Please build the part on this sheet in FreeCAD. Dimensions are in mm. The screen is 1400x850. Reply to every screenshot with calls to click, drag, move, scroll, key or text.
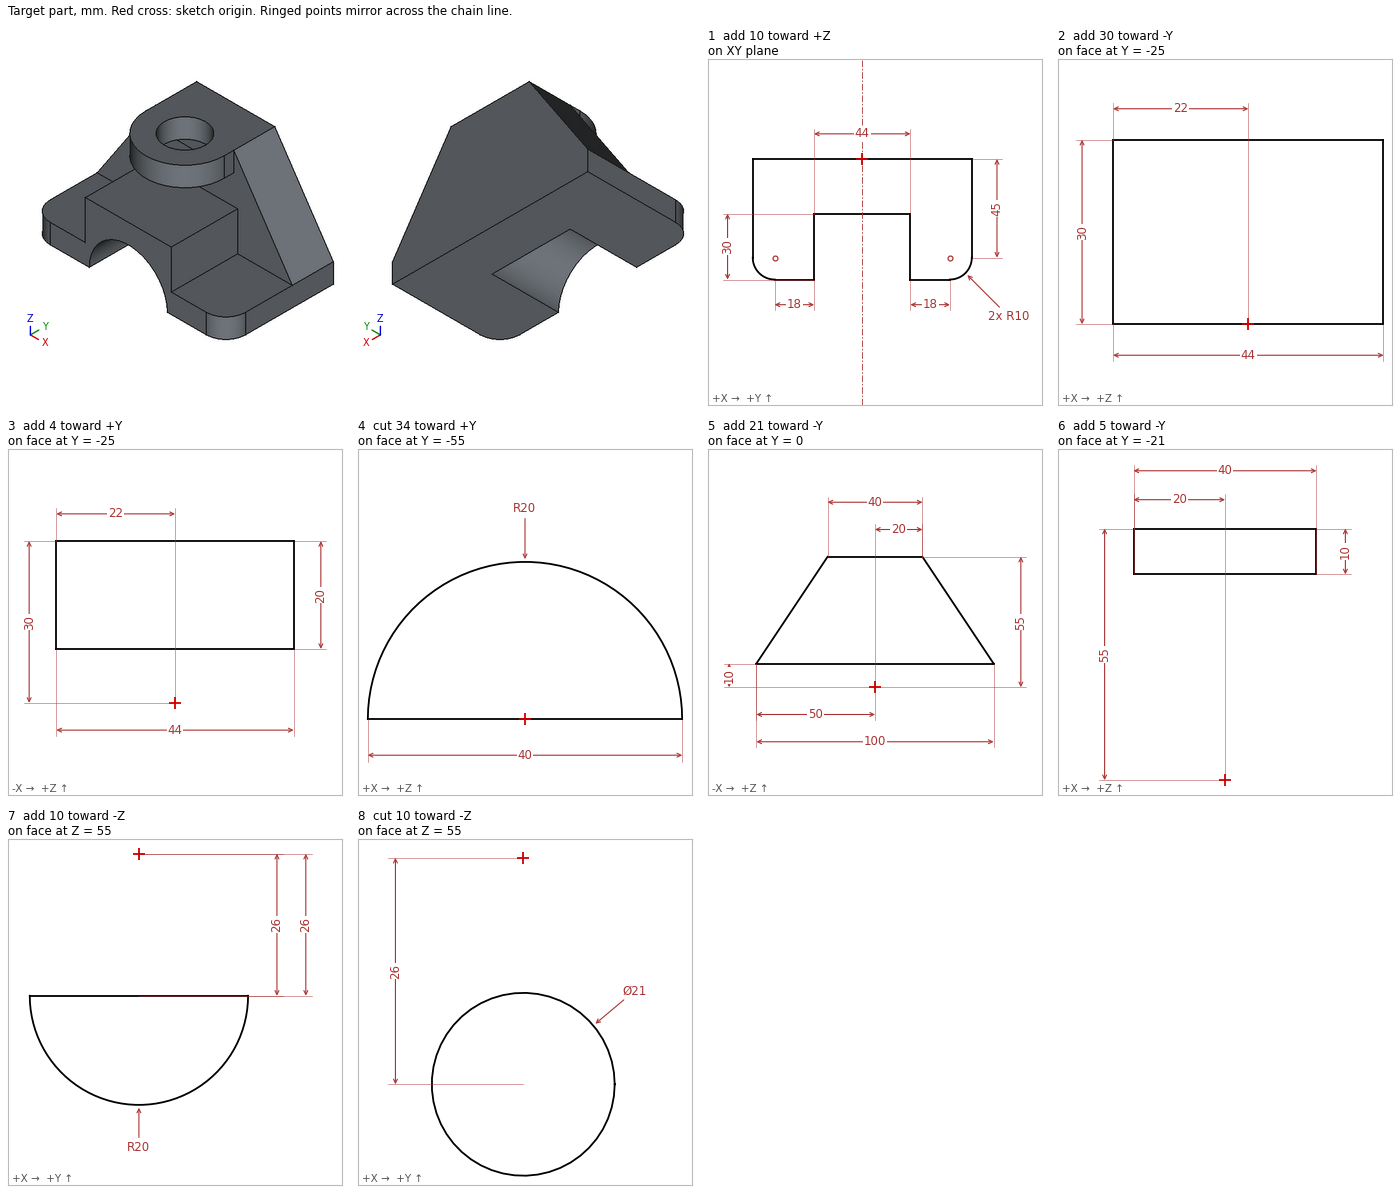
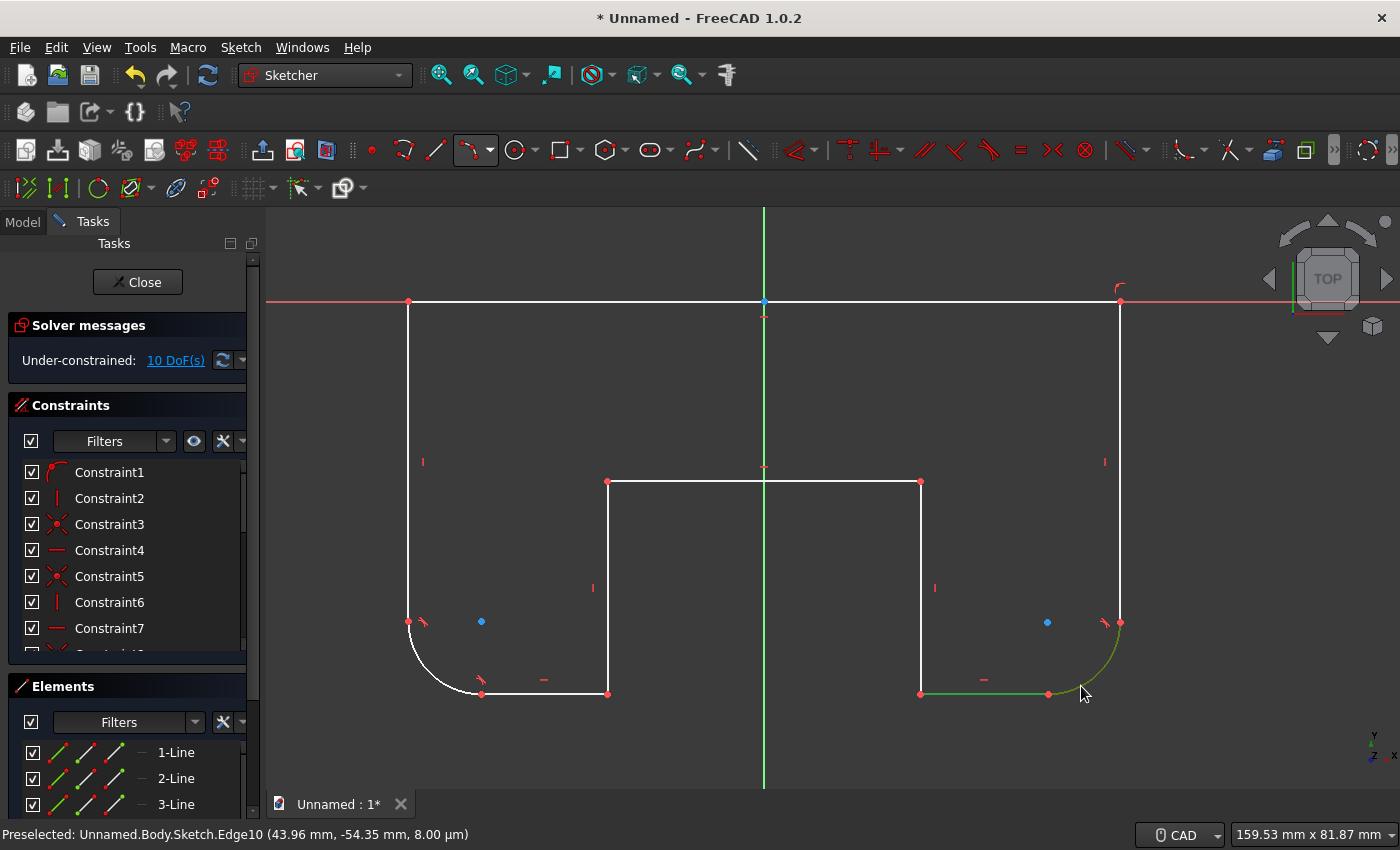
click(990, 150)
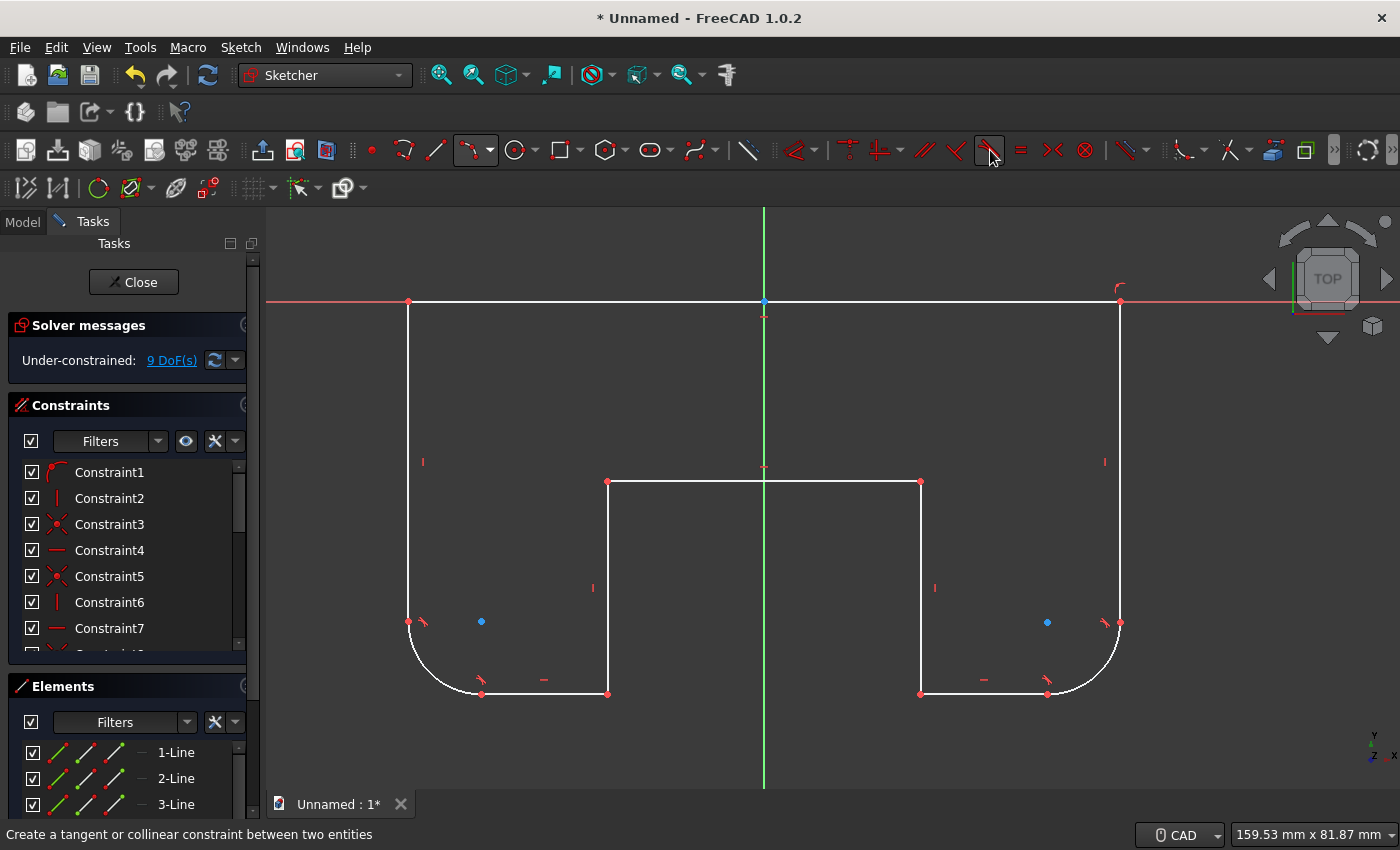
click(416, 654)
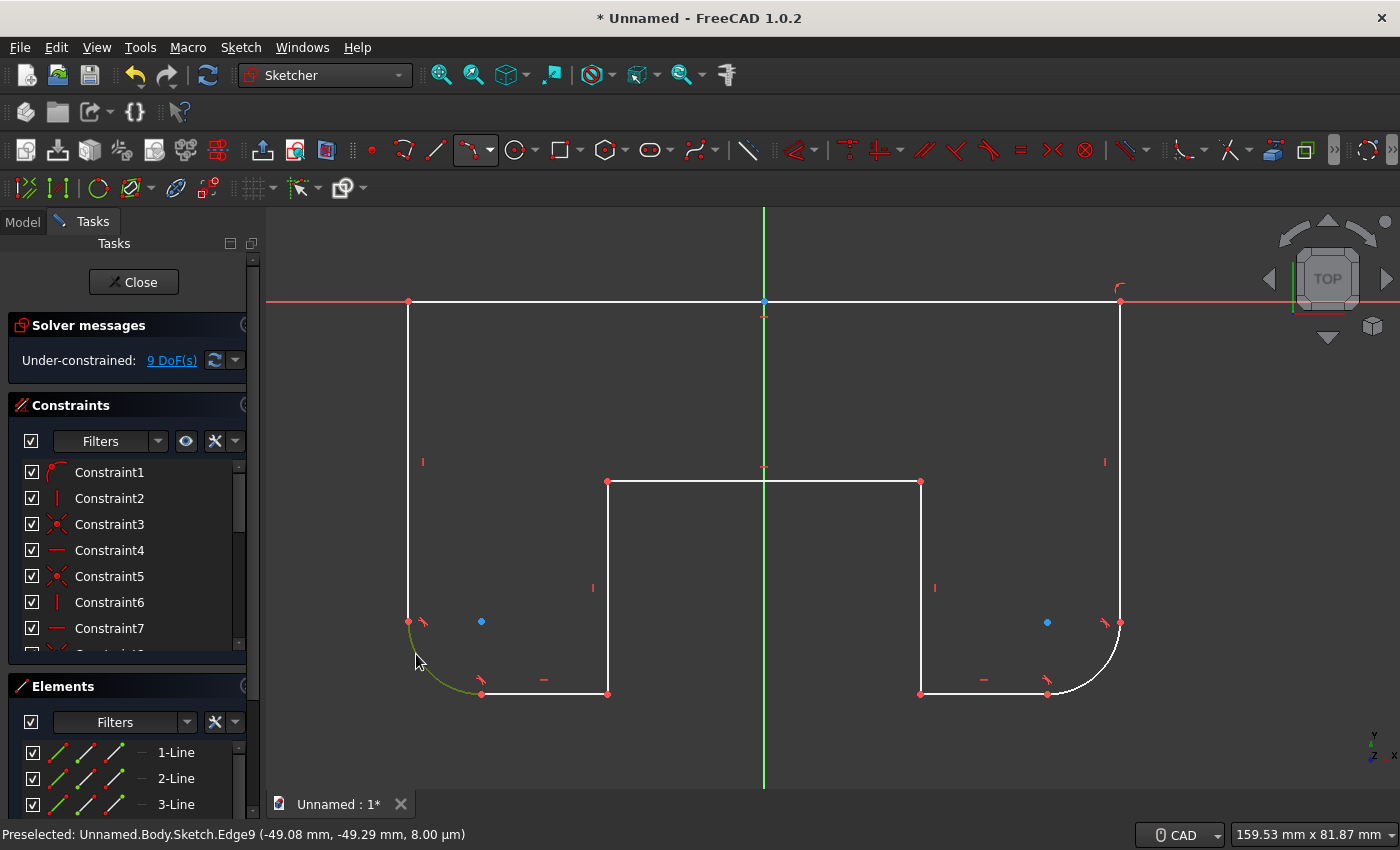
click(1081, 686)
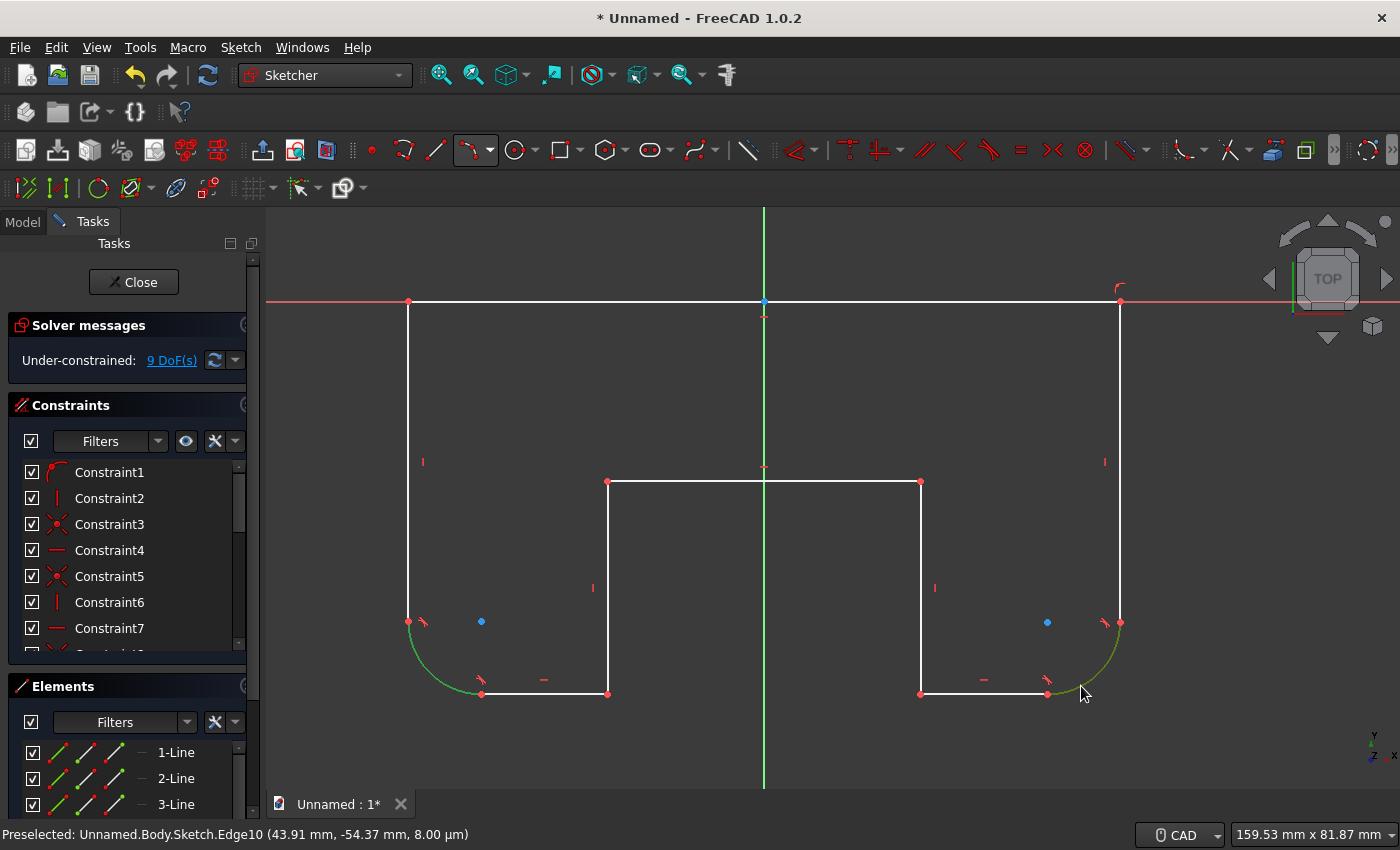
click(1022, 150)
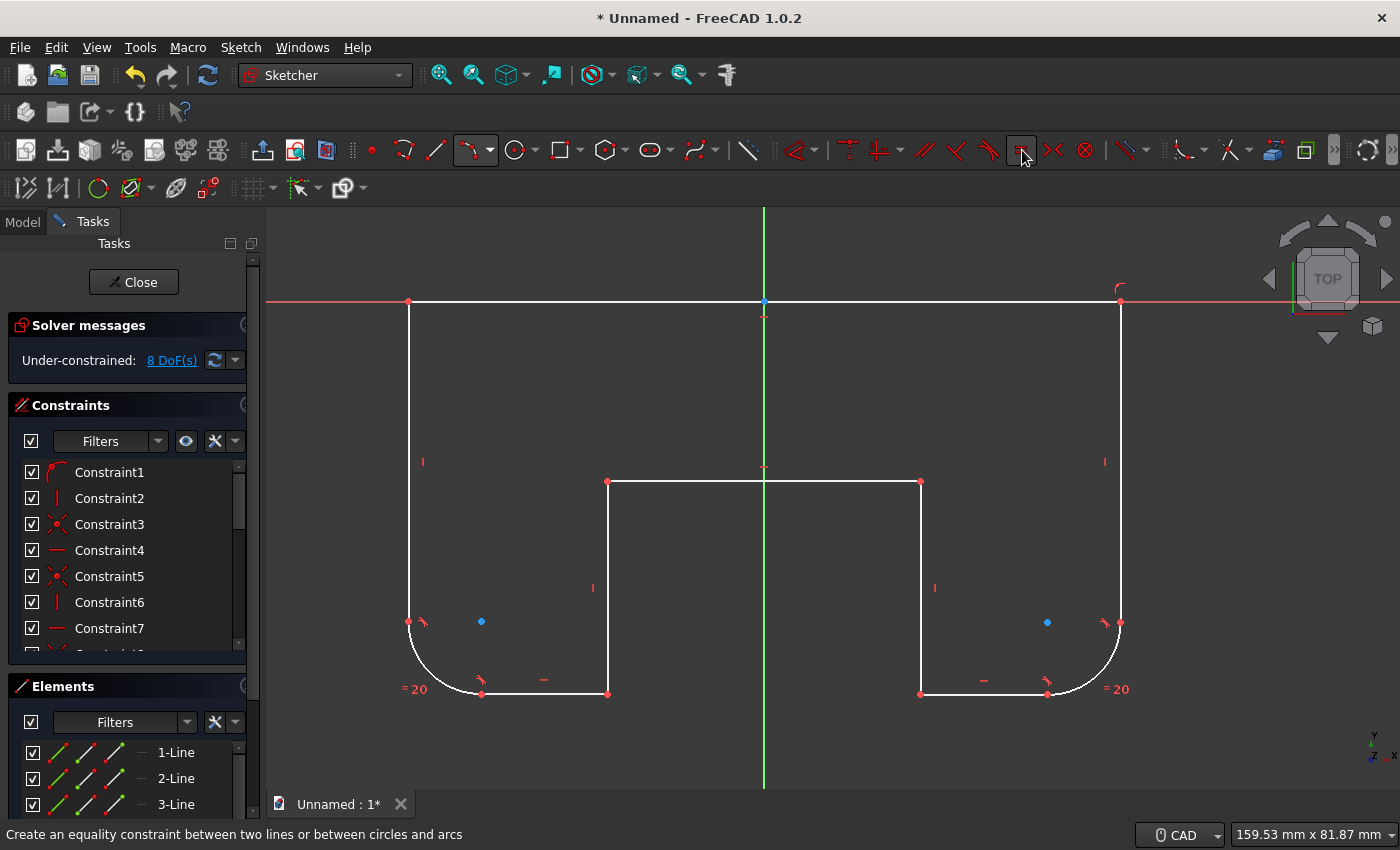
click(481, 621)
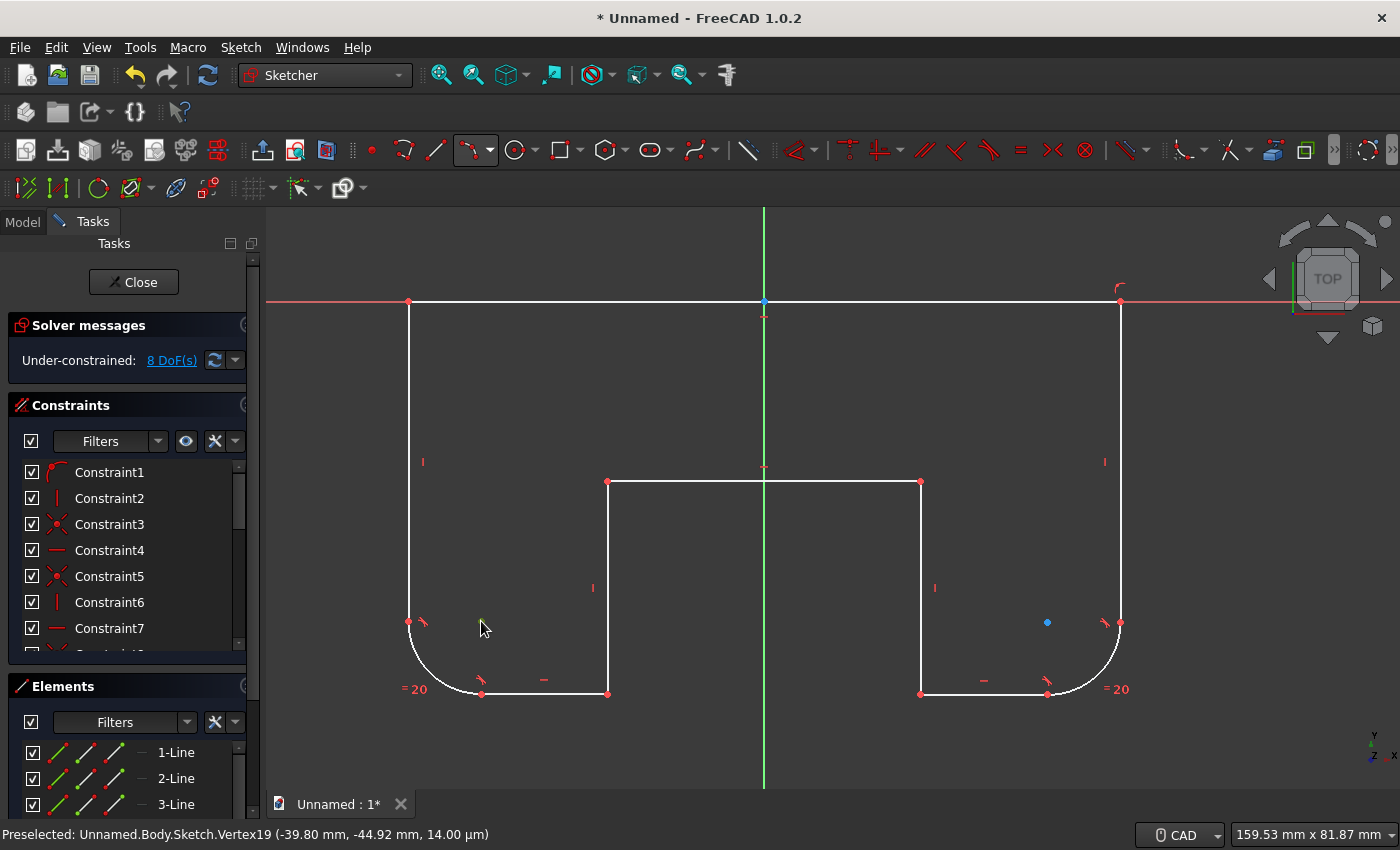
click(1048, 622)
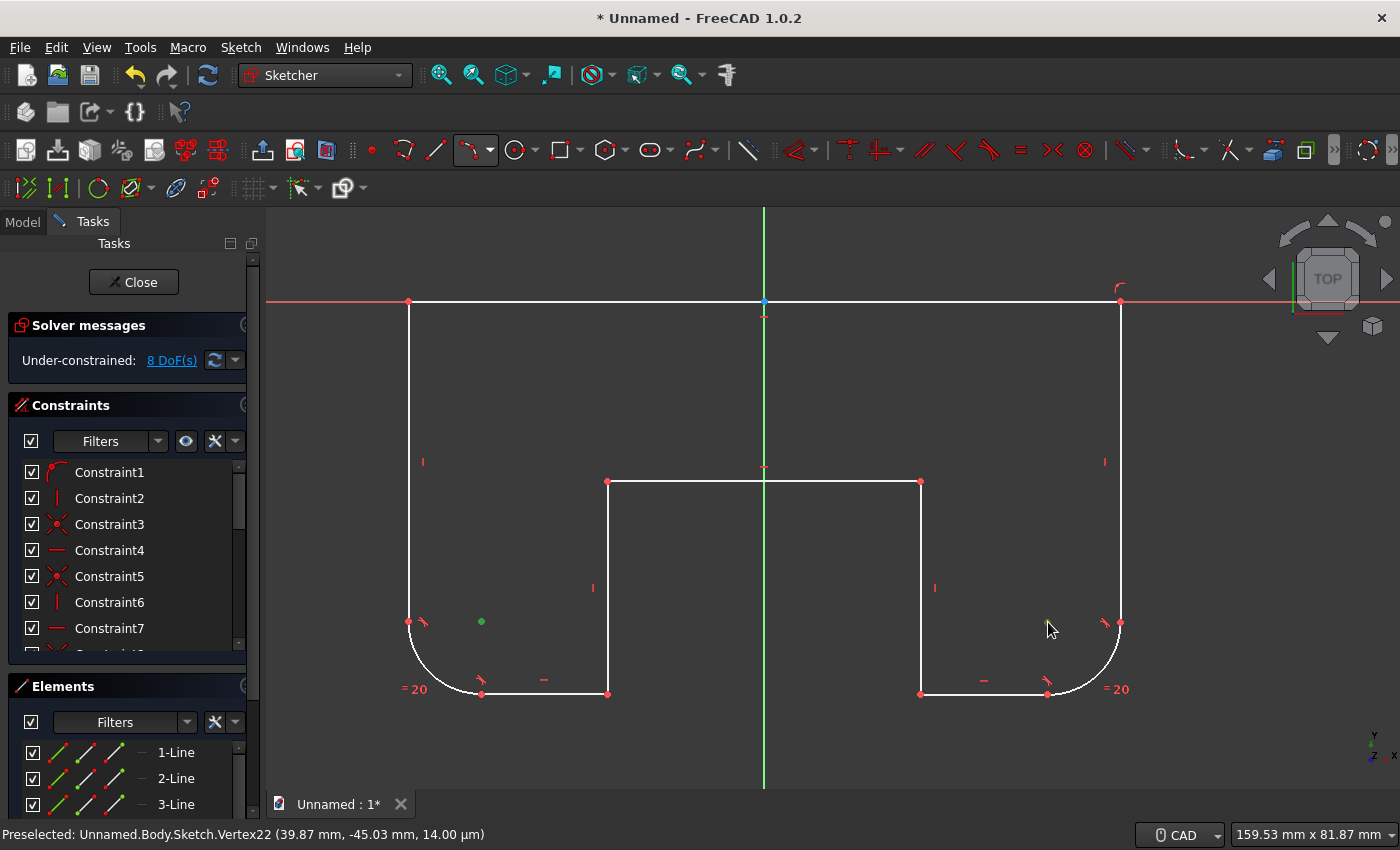
click(764, 723)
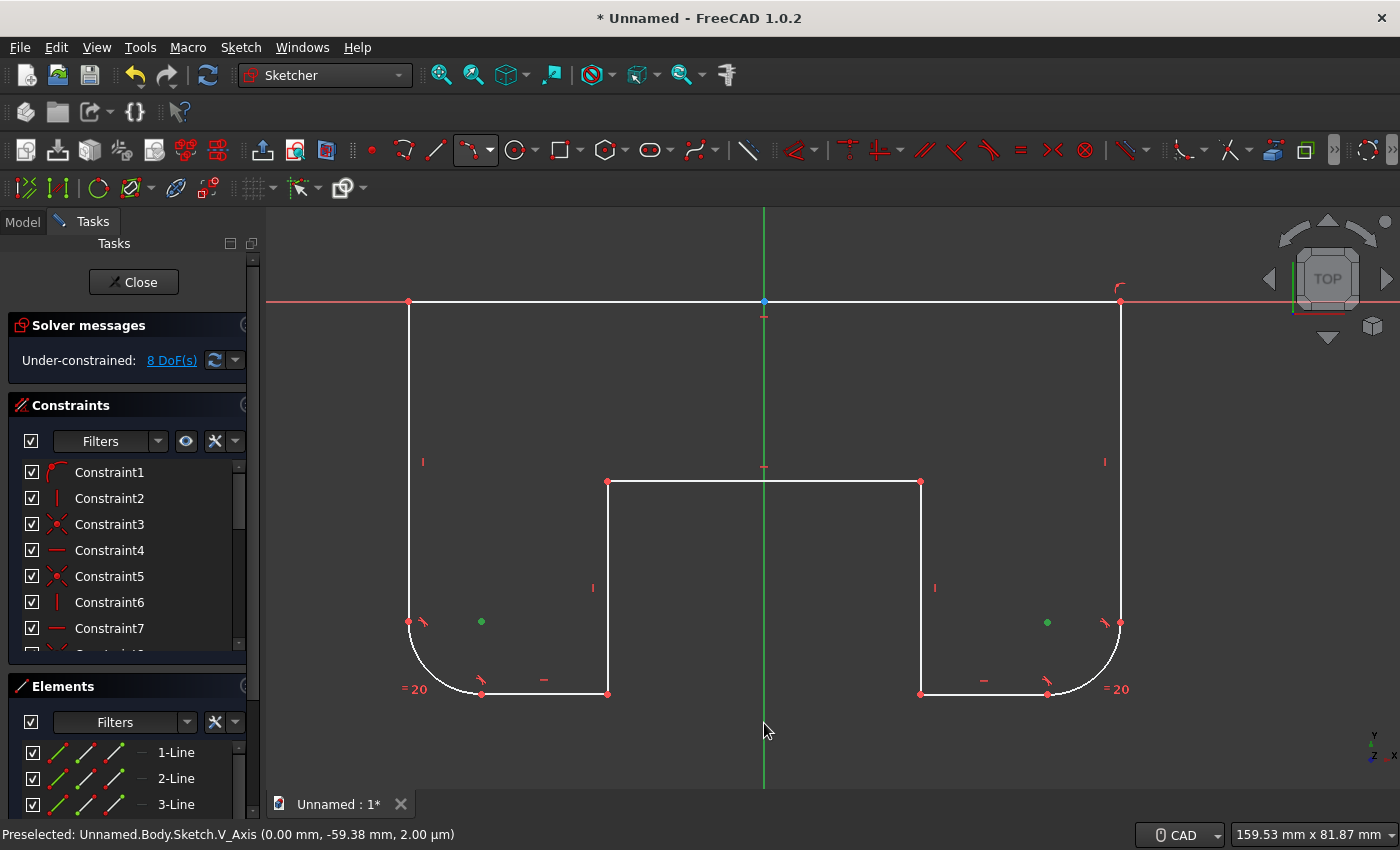
click(1054, 150)